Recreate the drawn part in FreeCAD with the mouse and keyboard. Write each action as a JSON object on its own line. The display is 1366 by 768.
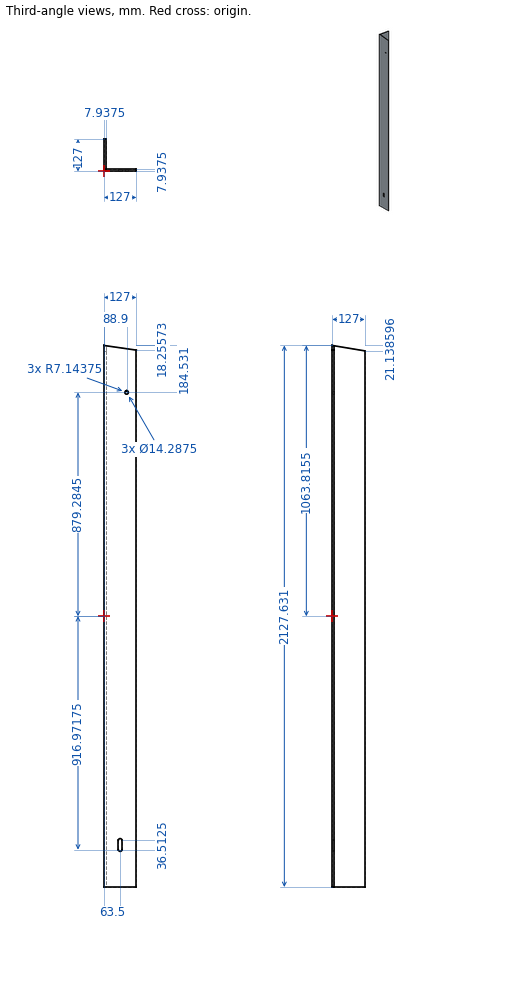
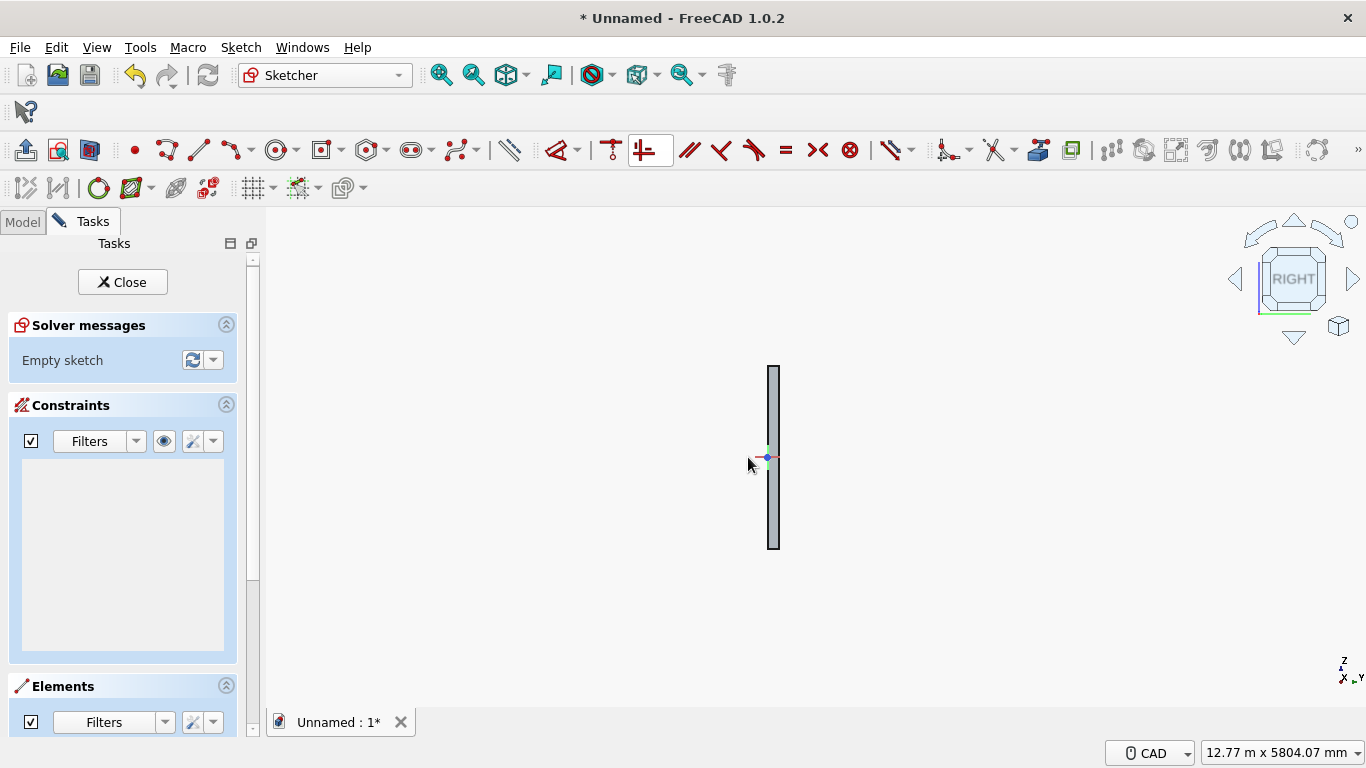
{"action": "scroll", "coordinate": [775, 362], "scroll_direction": "up", "scroll_amount": 15}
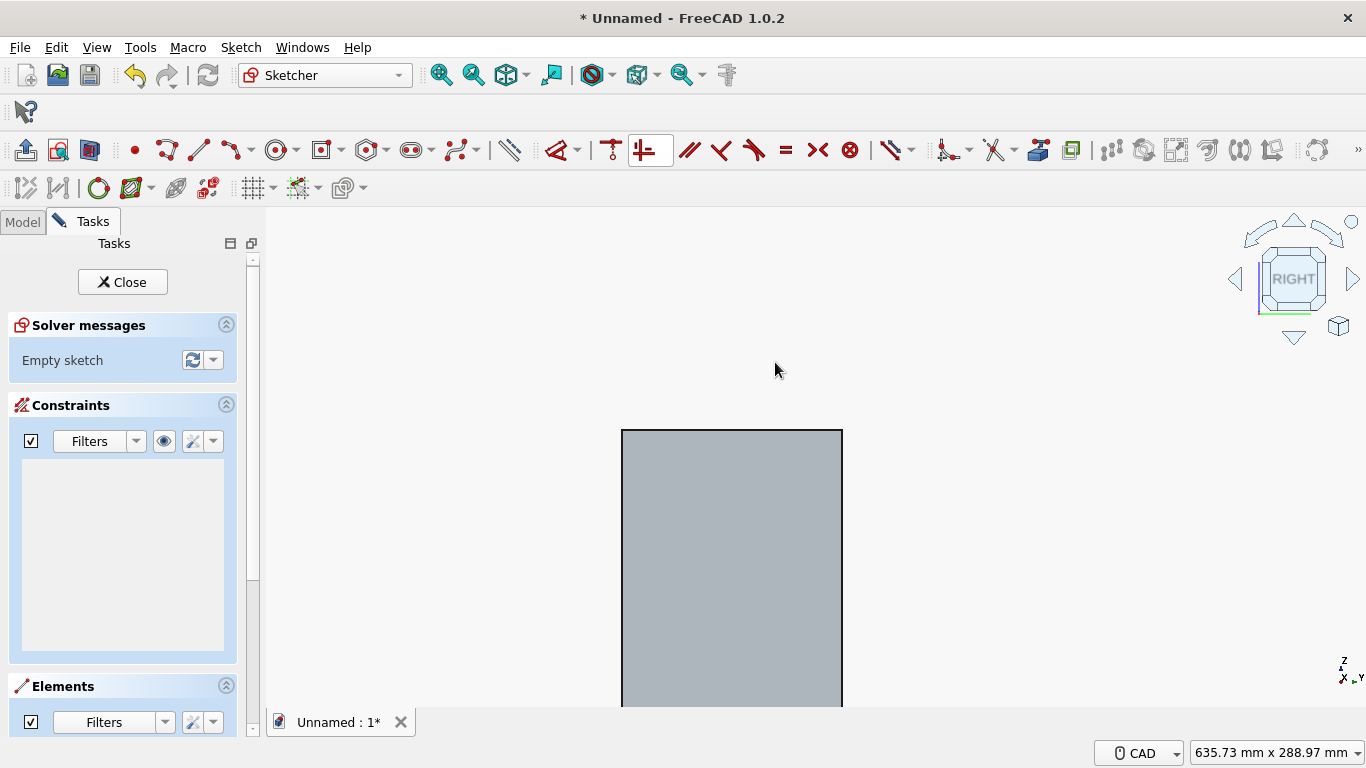
{"action": "scroll", "coordinate": [723, 443], "scroll_direction": "up", "scroll_amount": 5}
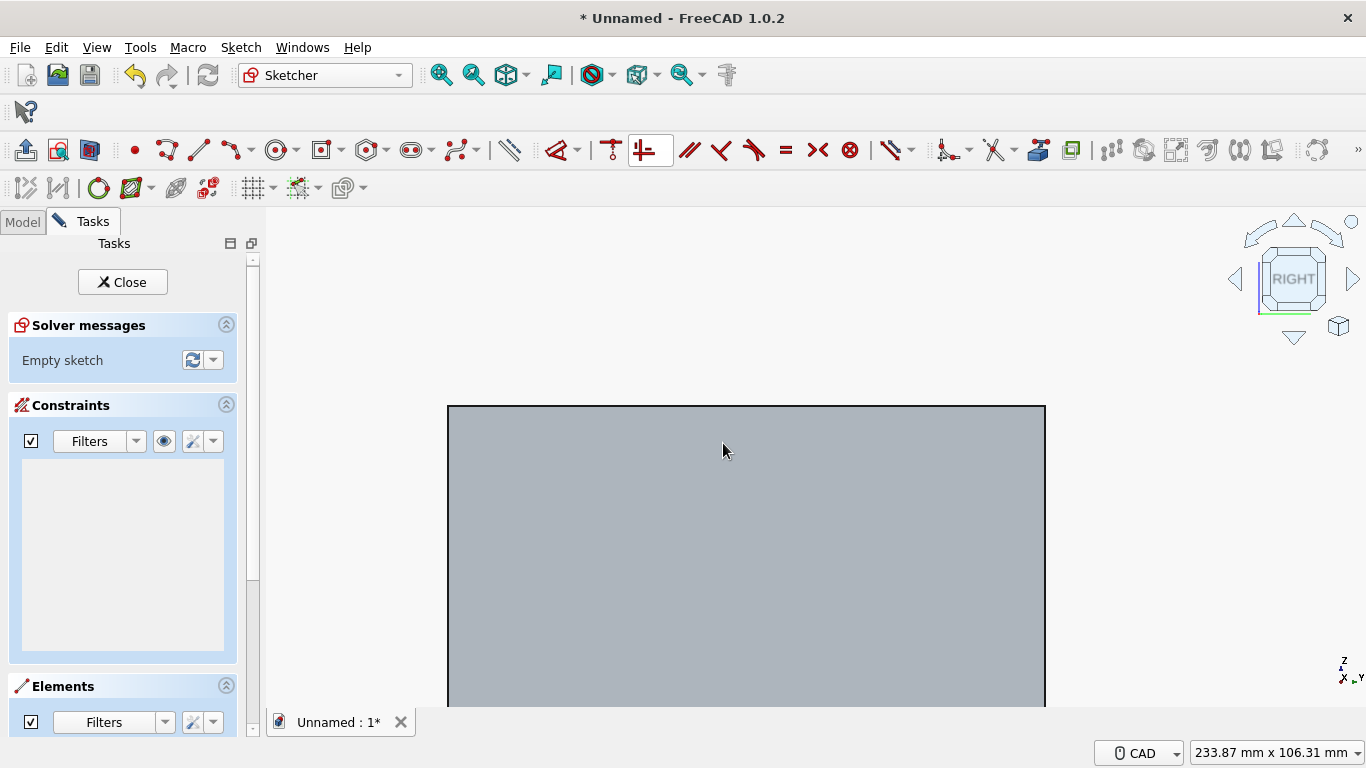
{"action": "key", "text": "g m"}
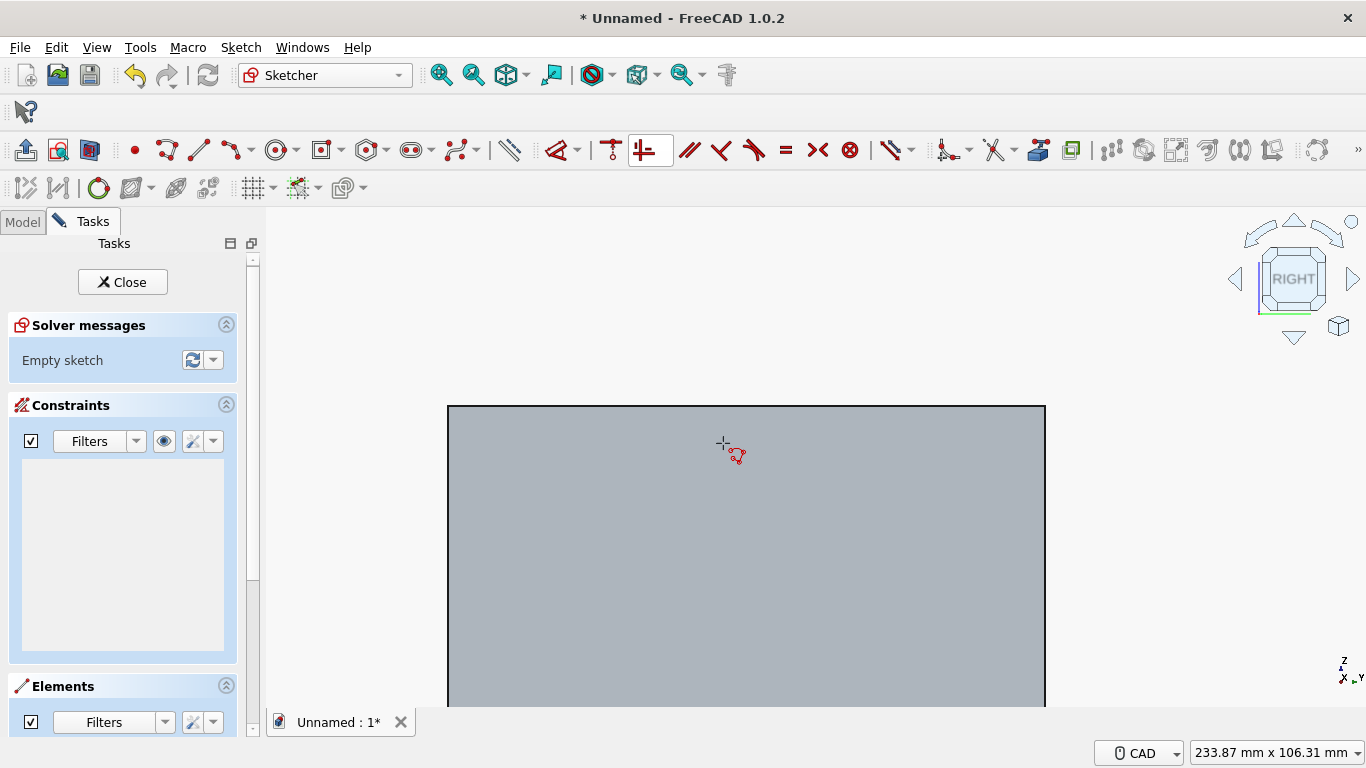
{"action": "left_click", "coordinate": [1045, 506]}
{"action": "left_click", "coordinate": [448, 406]}
{"action": "left_click", "coordinate": [1045, 406]}
{"action": "left_click", "coordinate": [1045, 507]}
{"action": "key", "text": "Escape"}
{"action": "key", "text": "Escape"}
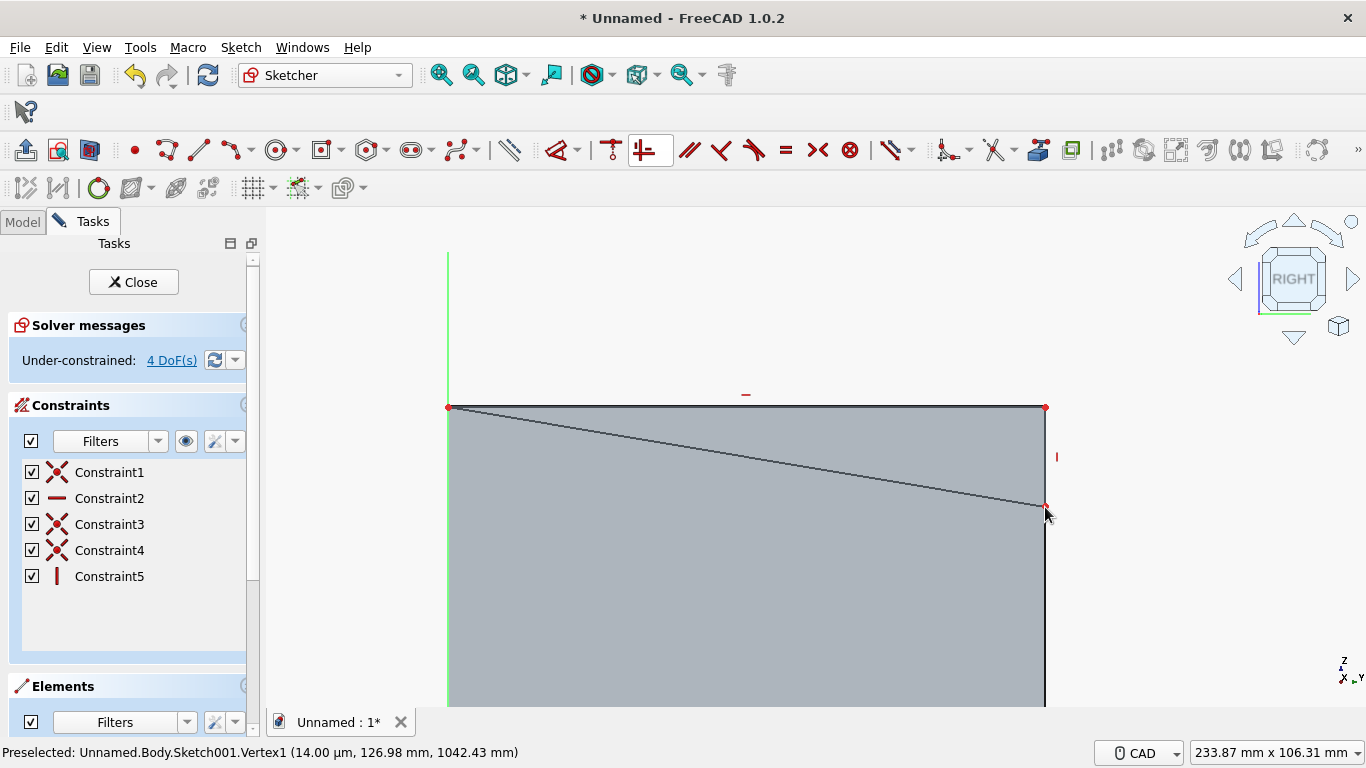
{"action": "left_click", "coordinate": [448, 407]}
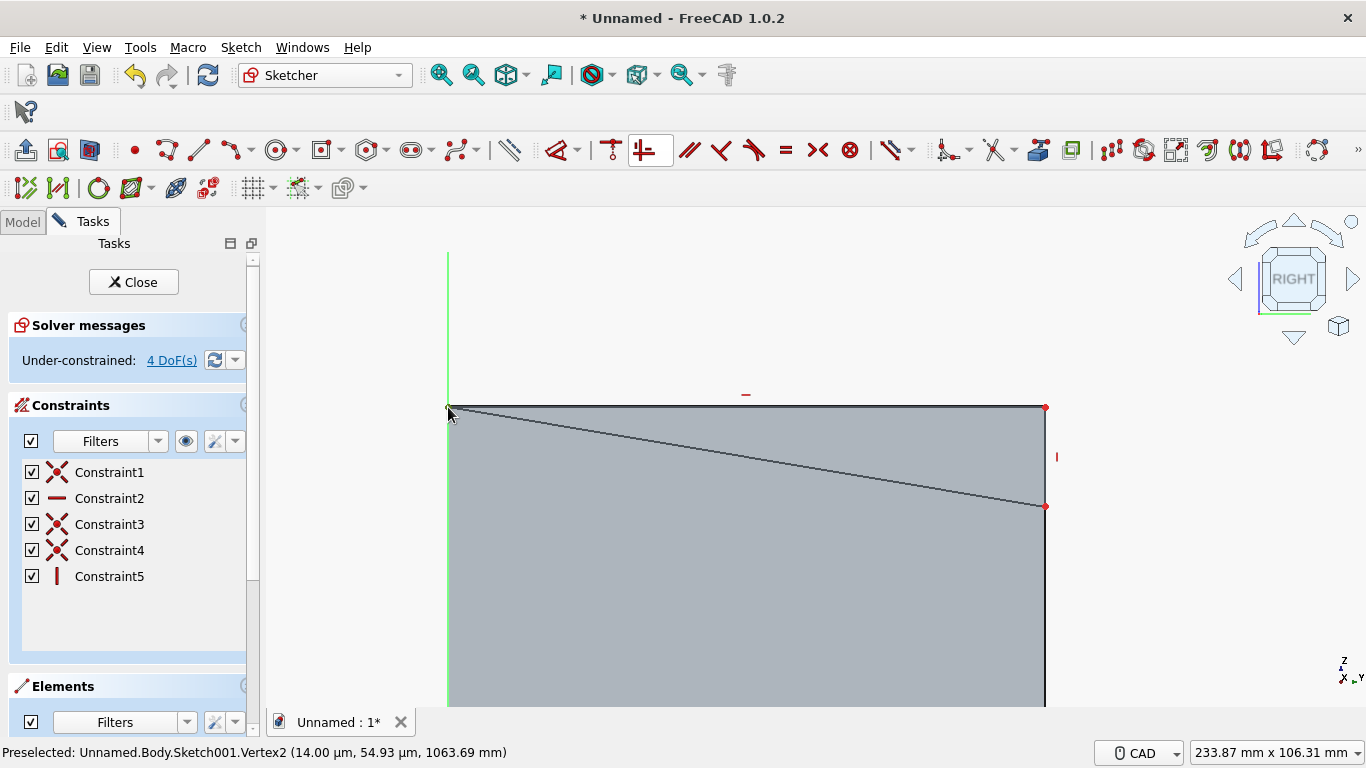
{"action": "left_click", "coordinate": [448, 647]}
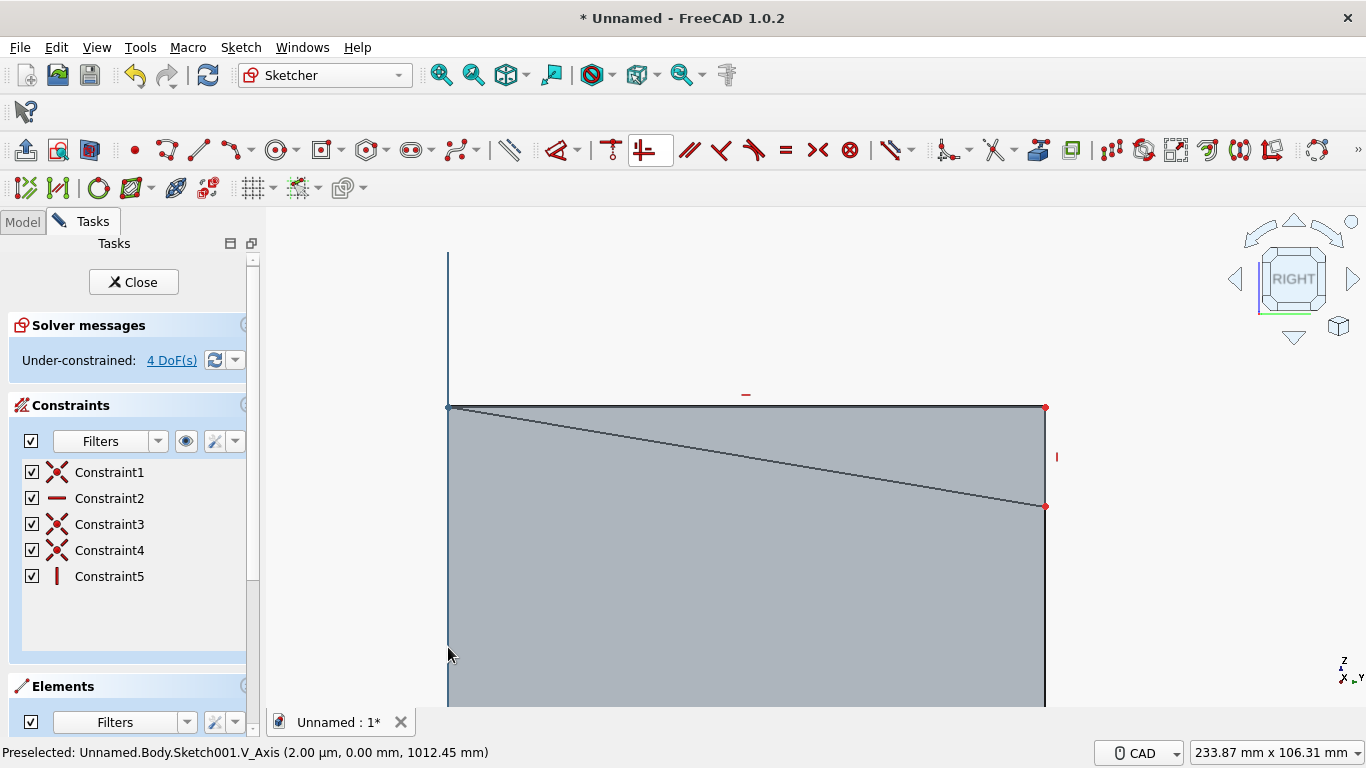
{"action": "key", "text": "c"}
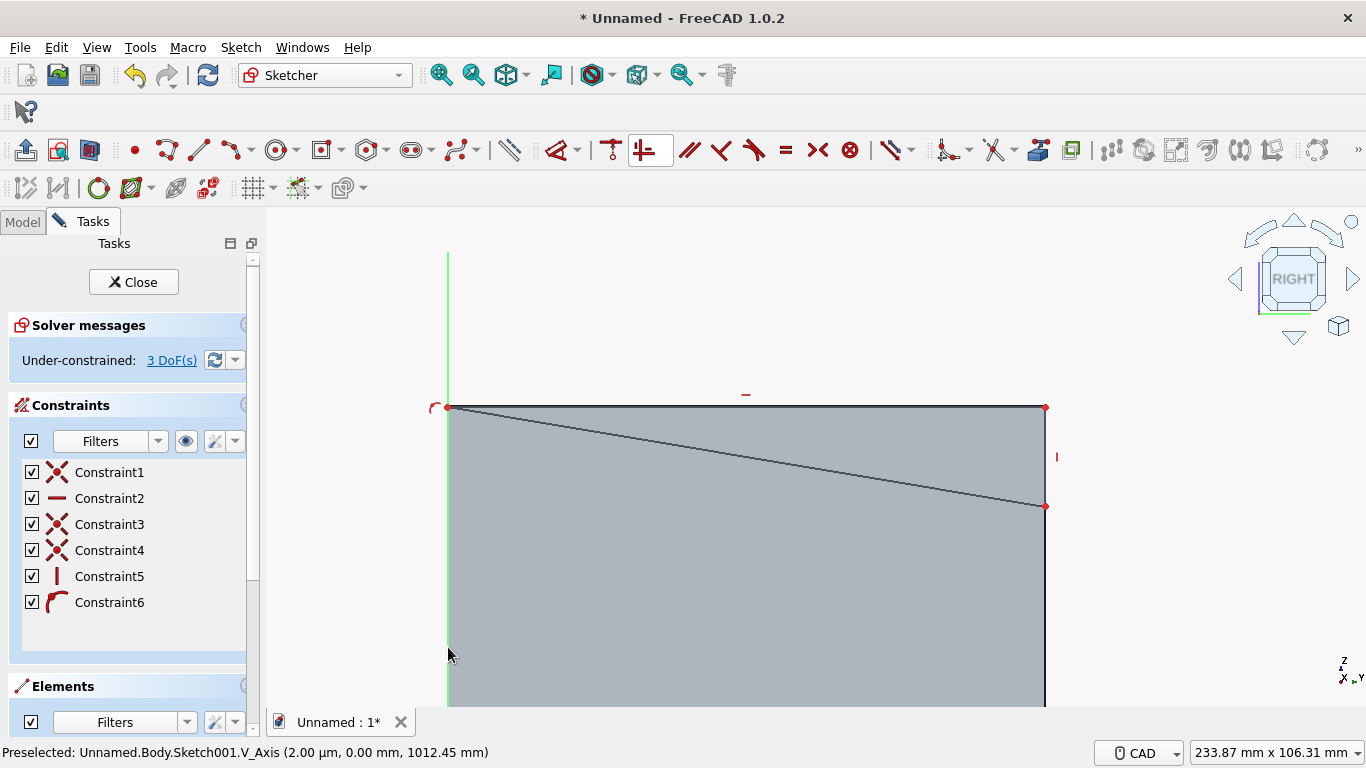
{"action": "key", "text": "d"}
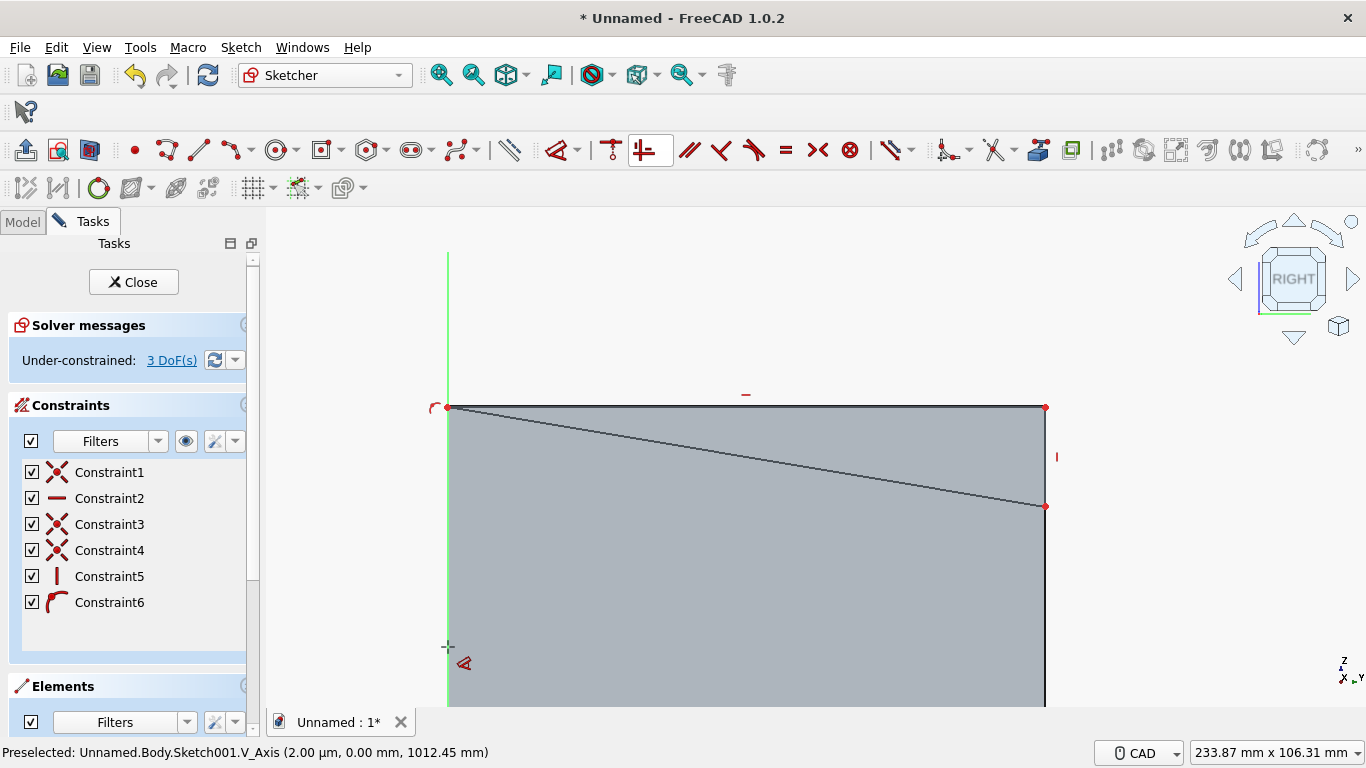
{"action": "left_click", "coordinate": [627, 407]}
{"action": "left_click", "coordinate": [746, 373]}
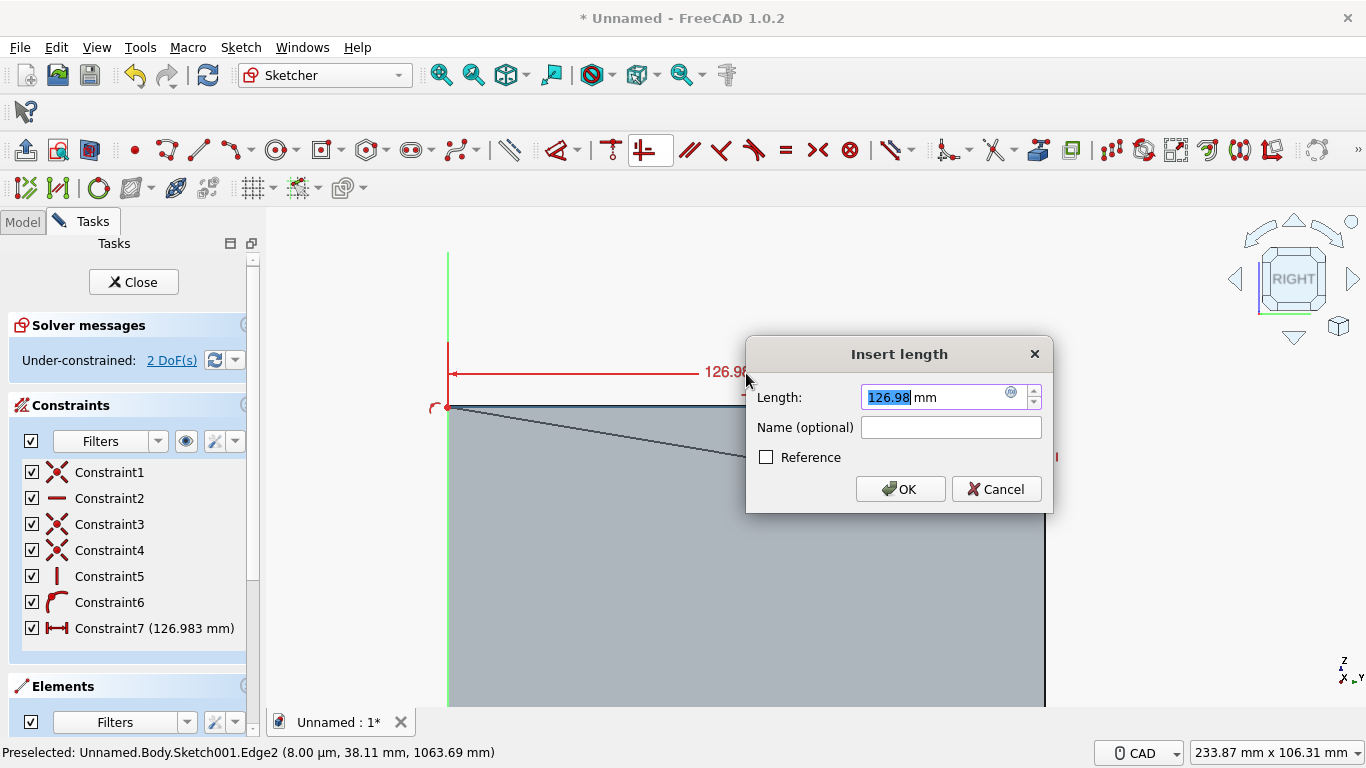
{"action": "type", "text": "127"}
{"action": "key", "text": "Return"}